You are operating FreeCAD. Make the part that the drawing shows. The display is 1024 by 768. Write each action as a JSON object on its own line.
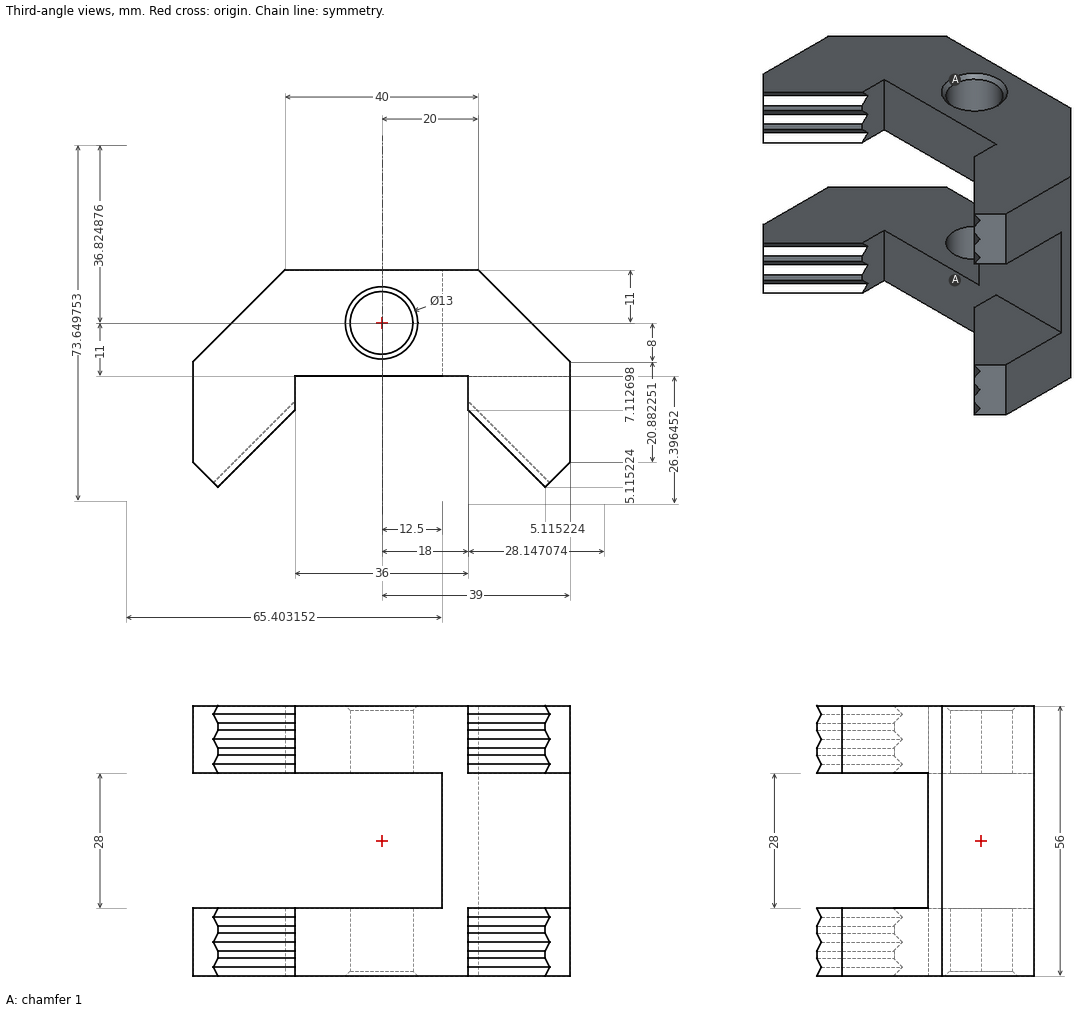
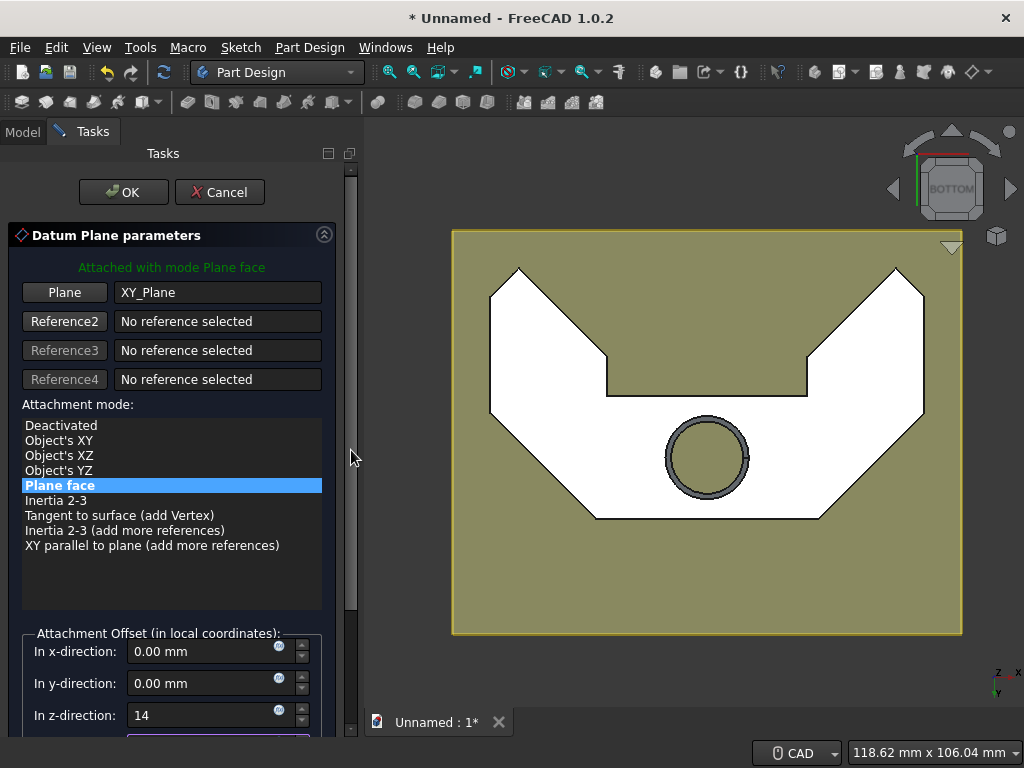
{"action": "left_click", "coordinate": [124, 192]}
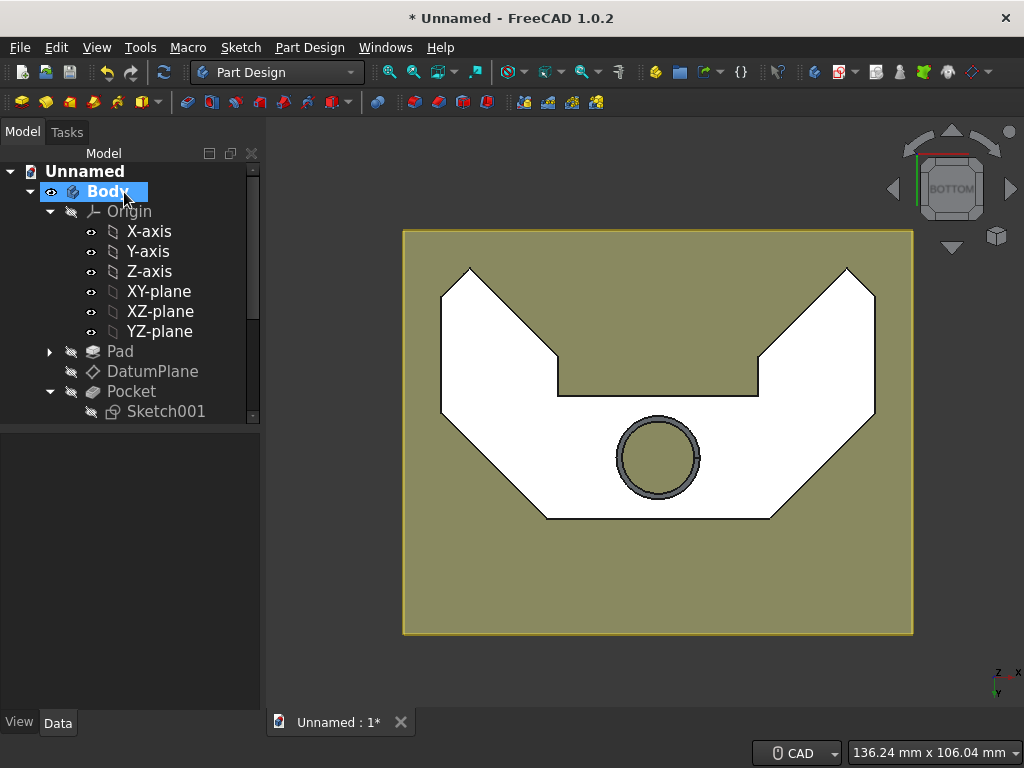
{"action": "scroll", "coordinate": [100, 287], "scroll_direction": "down", "scroll_amount": 3}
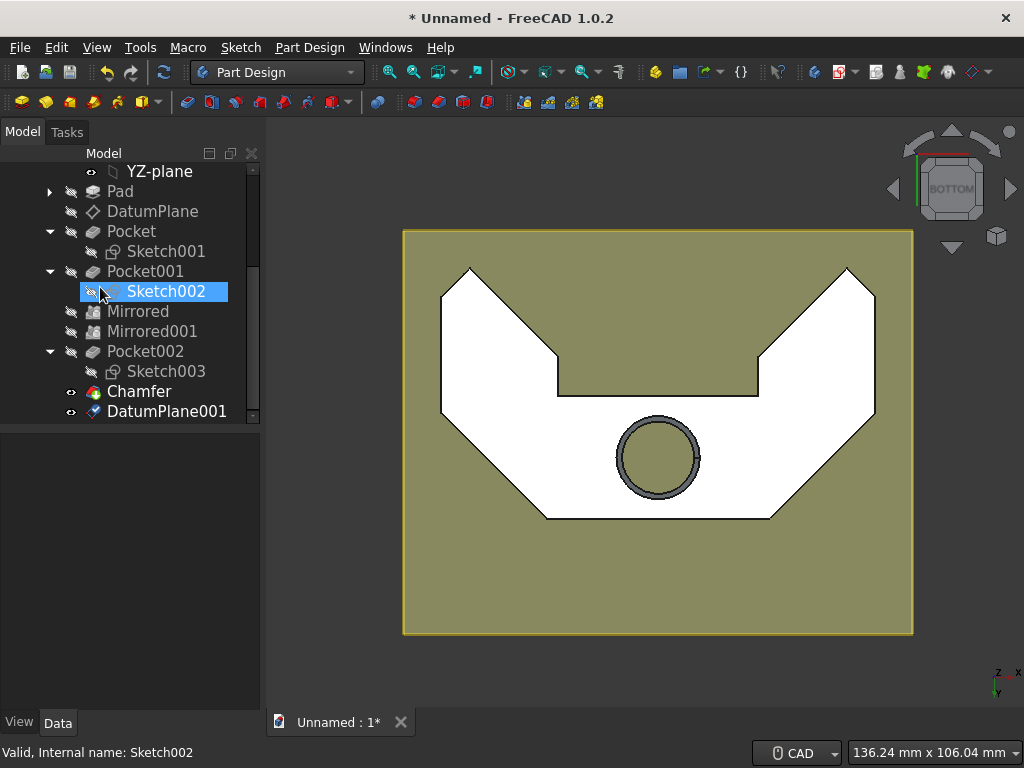
{"action": "left_click", "coordinate": [116, 412]}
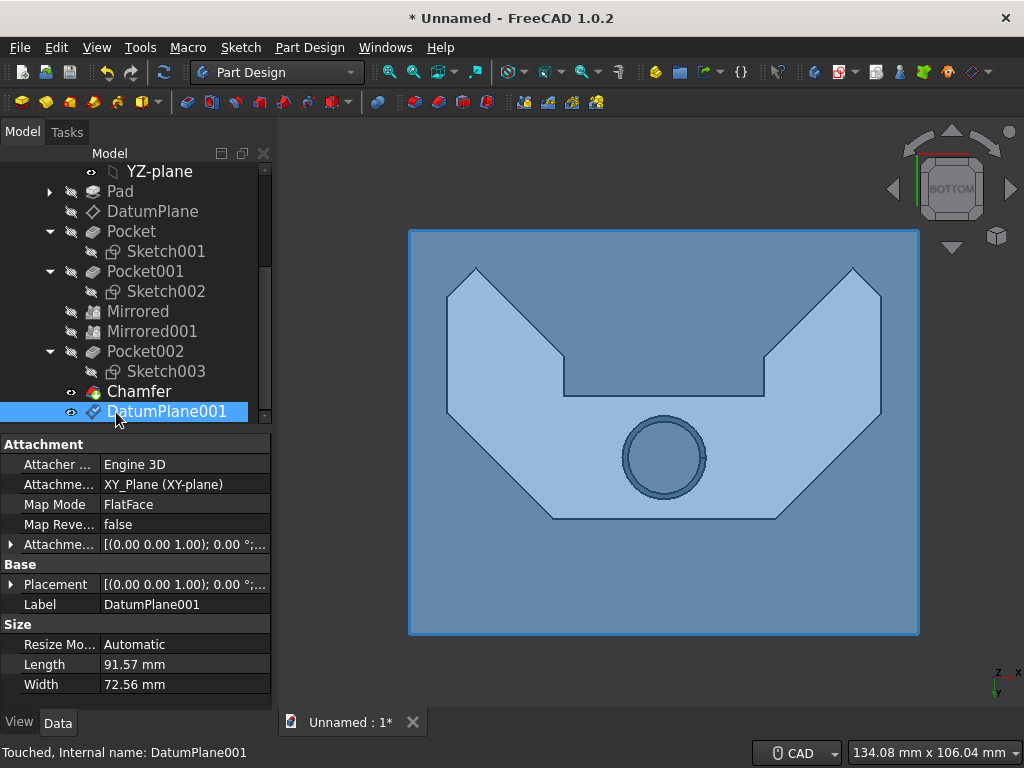
{"action": "left_click", "coordinate": [840, 72]}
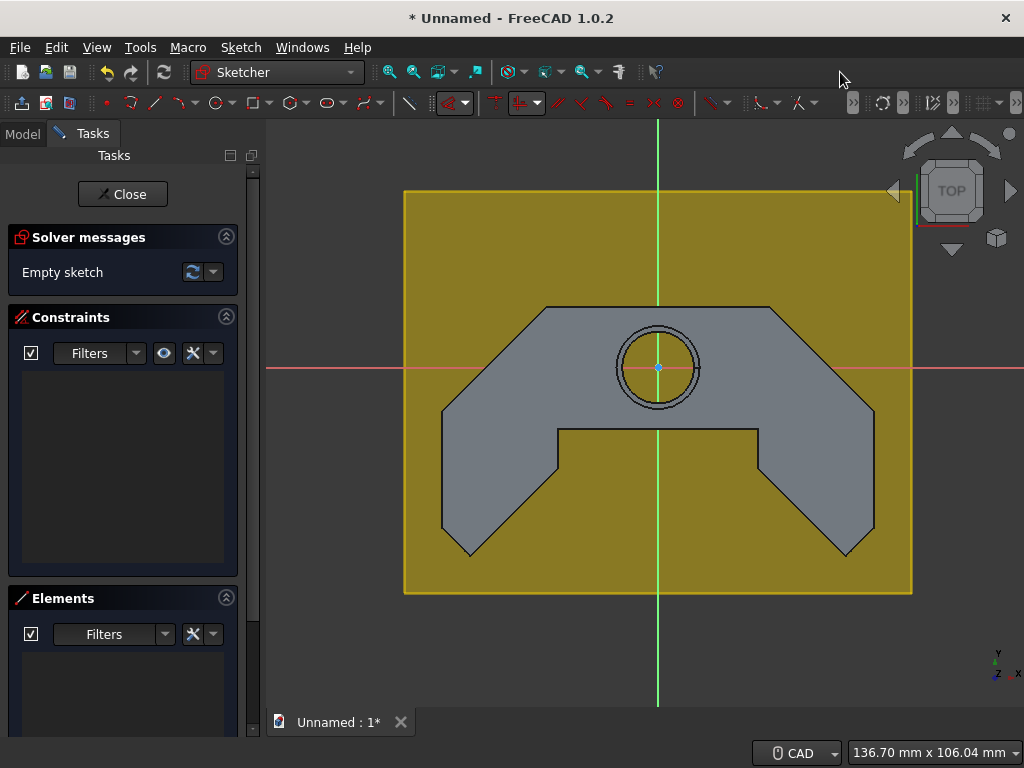
{"action": "left_click", "coordinate": [70, 104]}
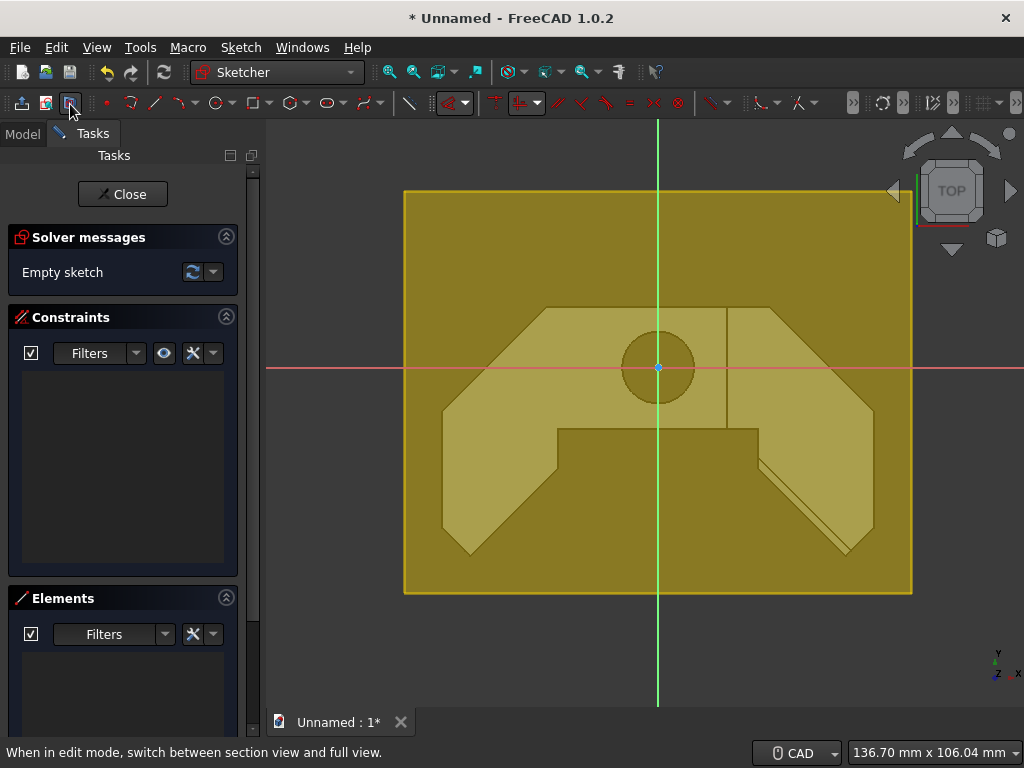
{"action": "scroll", "coordinate": [294, 150], "scroll_direction": "down", "scroll_amount": 1}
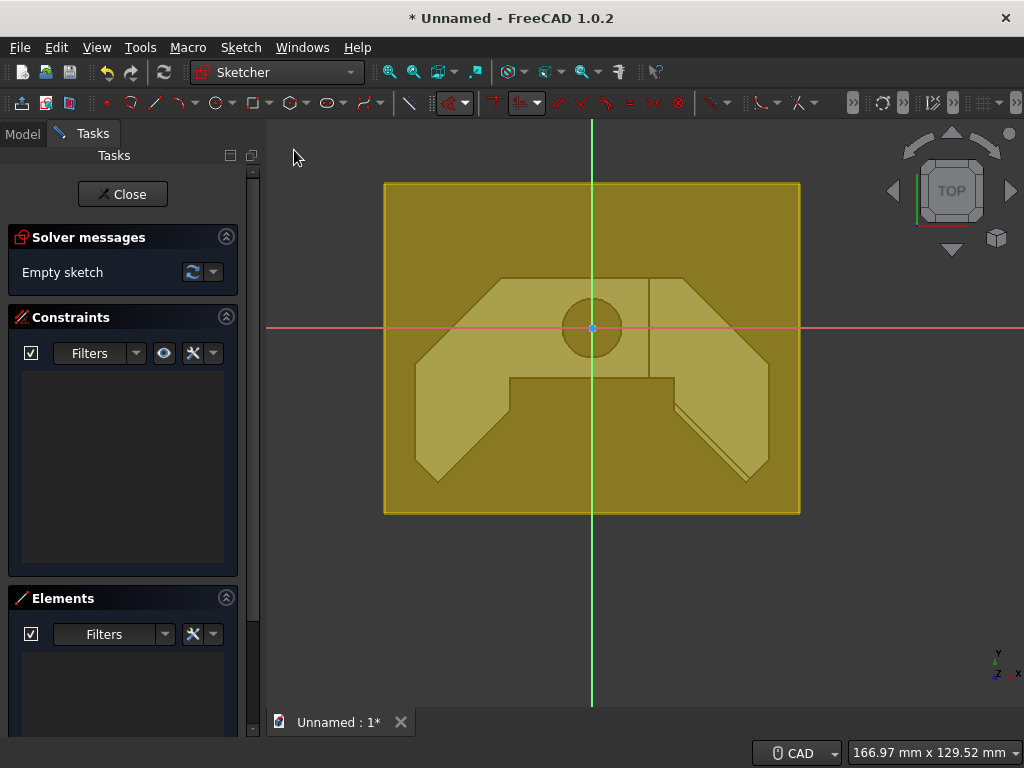
{"action": "scroll", "coordinate": [843, 413], "scroll_direction": "up", "scroll_amount": 3}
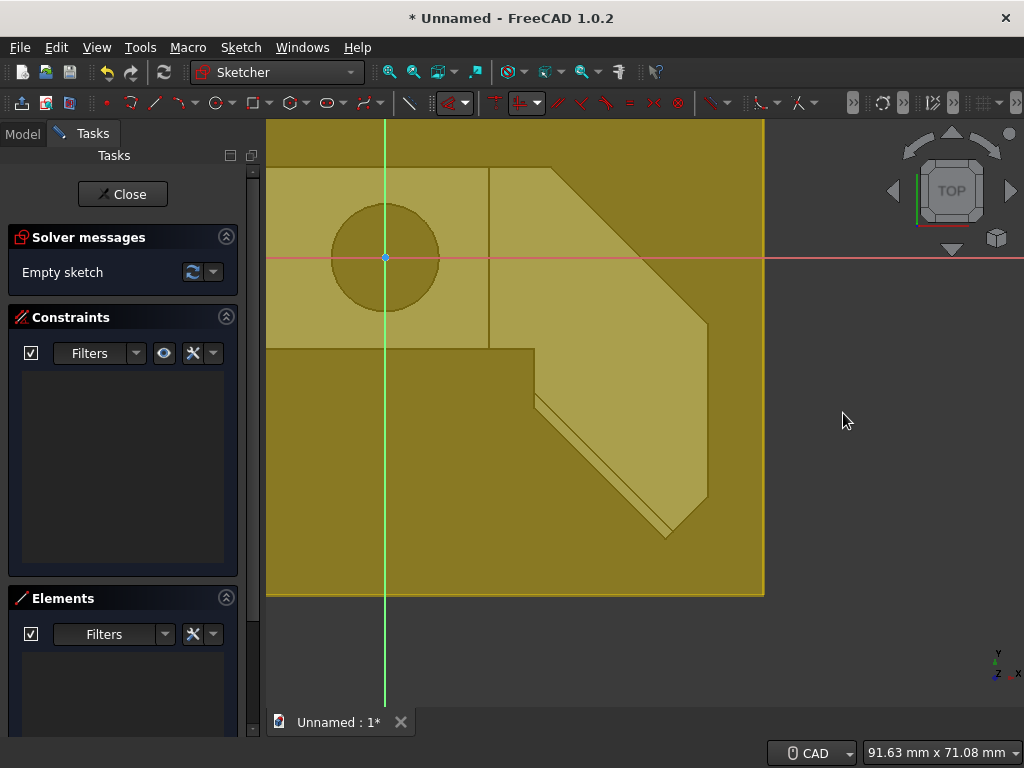
{"action": "key", "text": "g r"}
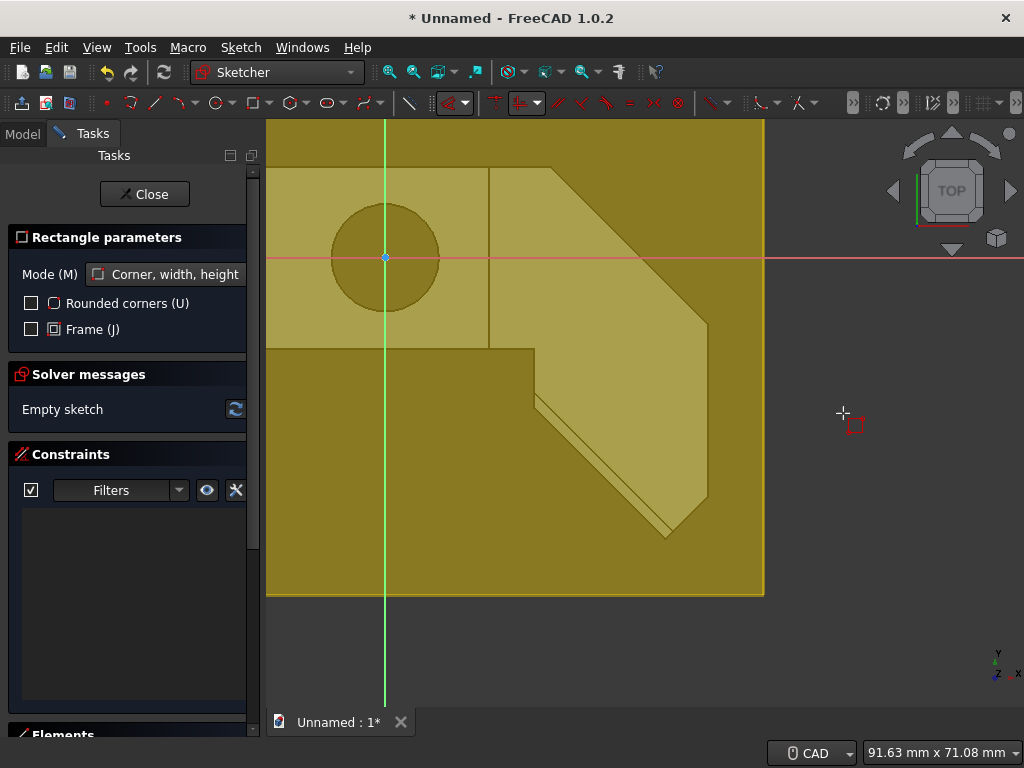
{"action": "left_click", "coordinate": [534, 349]}
{"action": "left_click", "coordinate": [767, 567]}
{"action": "key", "text": "Escape"}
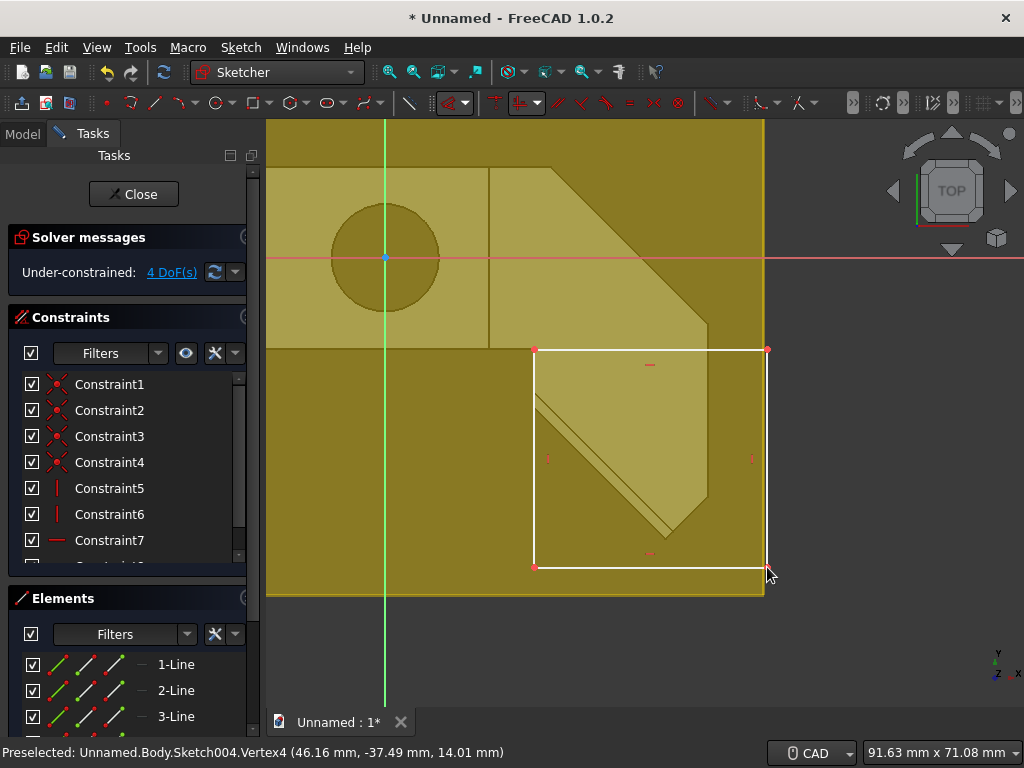
{"action": "left_click", "coordinate": [534, 350]}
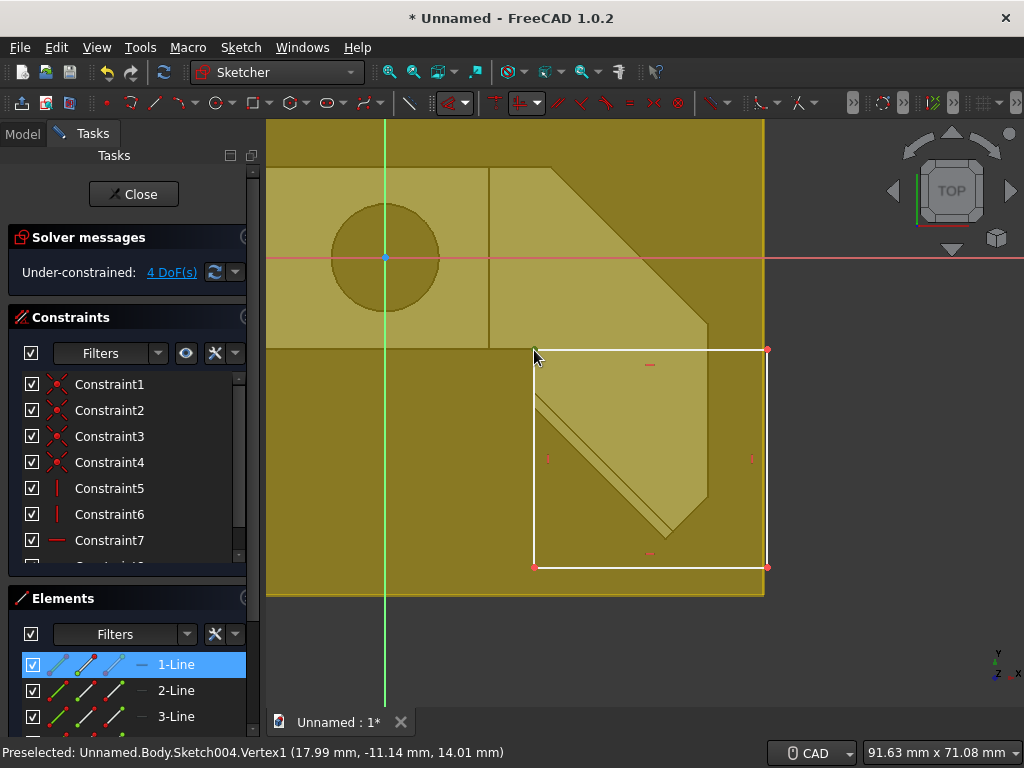
{"action": "key", "text": "l"}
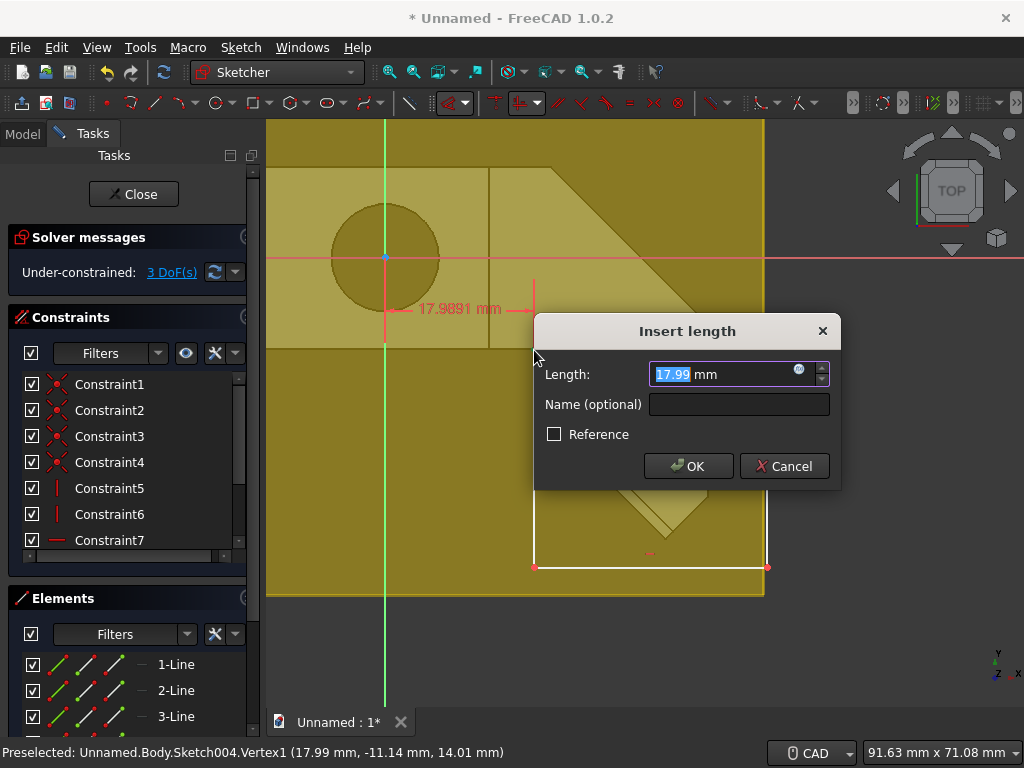
{"action": "type", "text": "18"}
{"action": "key", "text": "Return"}